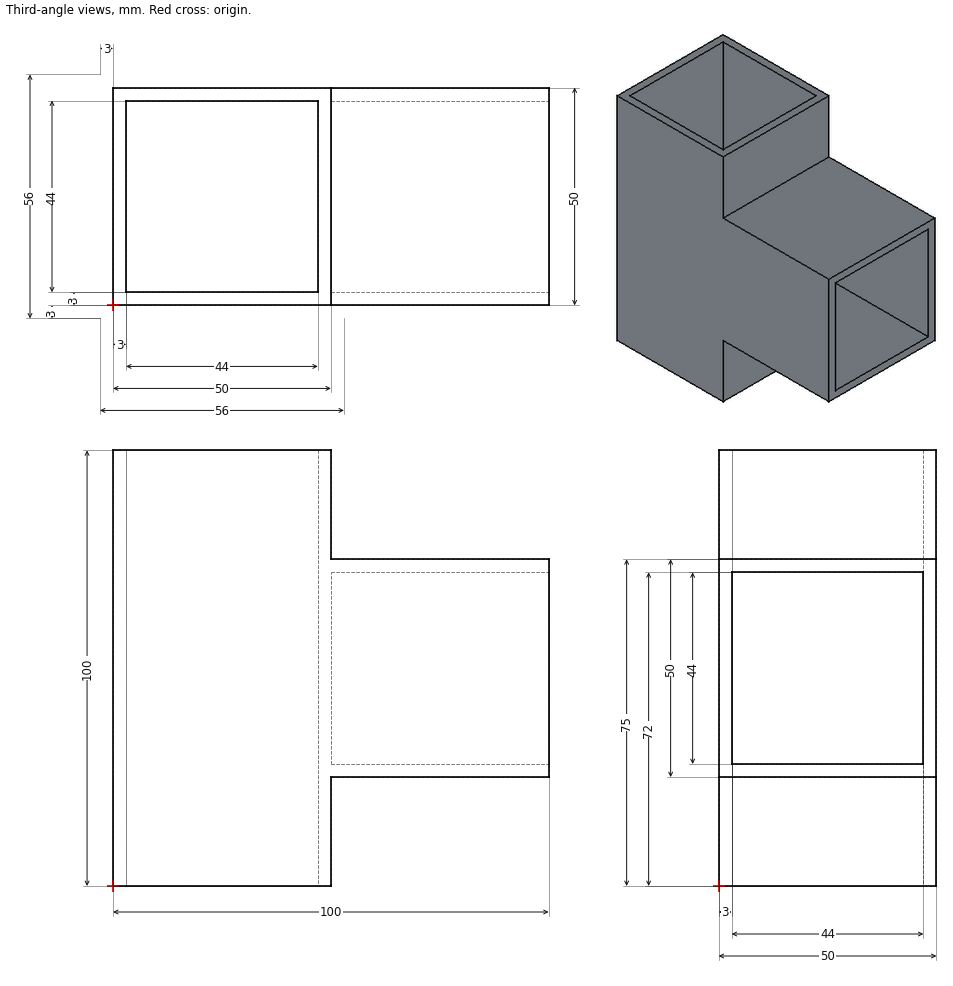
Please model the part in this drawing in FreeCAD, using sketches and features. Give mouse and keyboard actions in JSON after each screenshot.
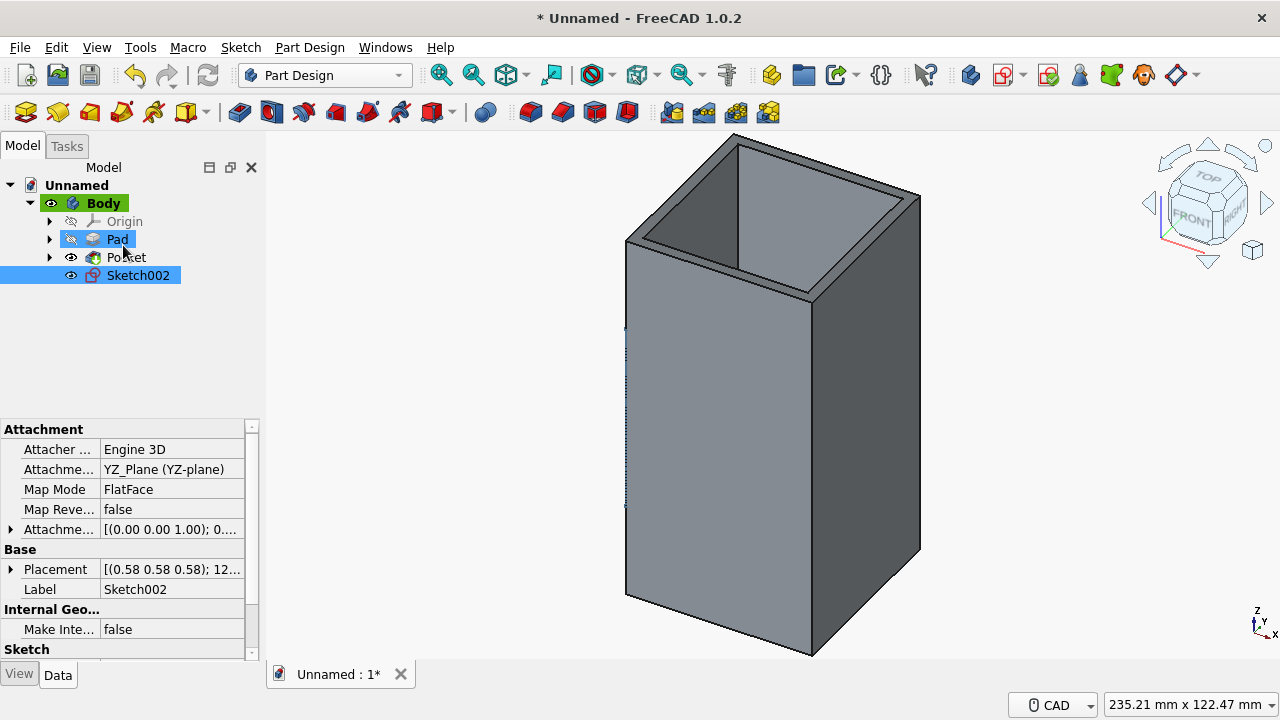
{"action": "left_click", "coordinate": [26, 112]}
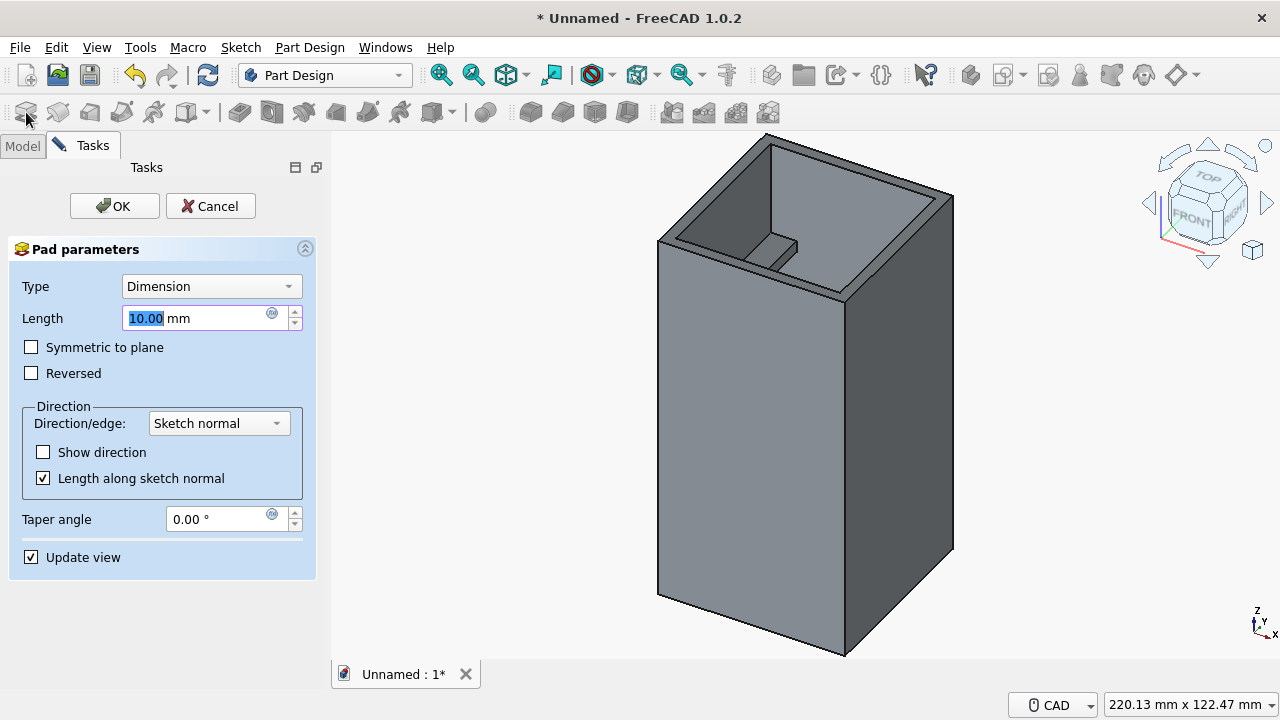
{"action": "type", "text": "100"}
{"action": "key", "text": "Tab"}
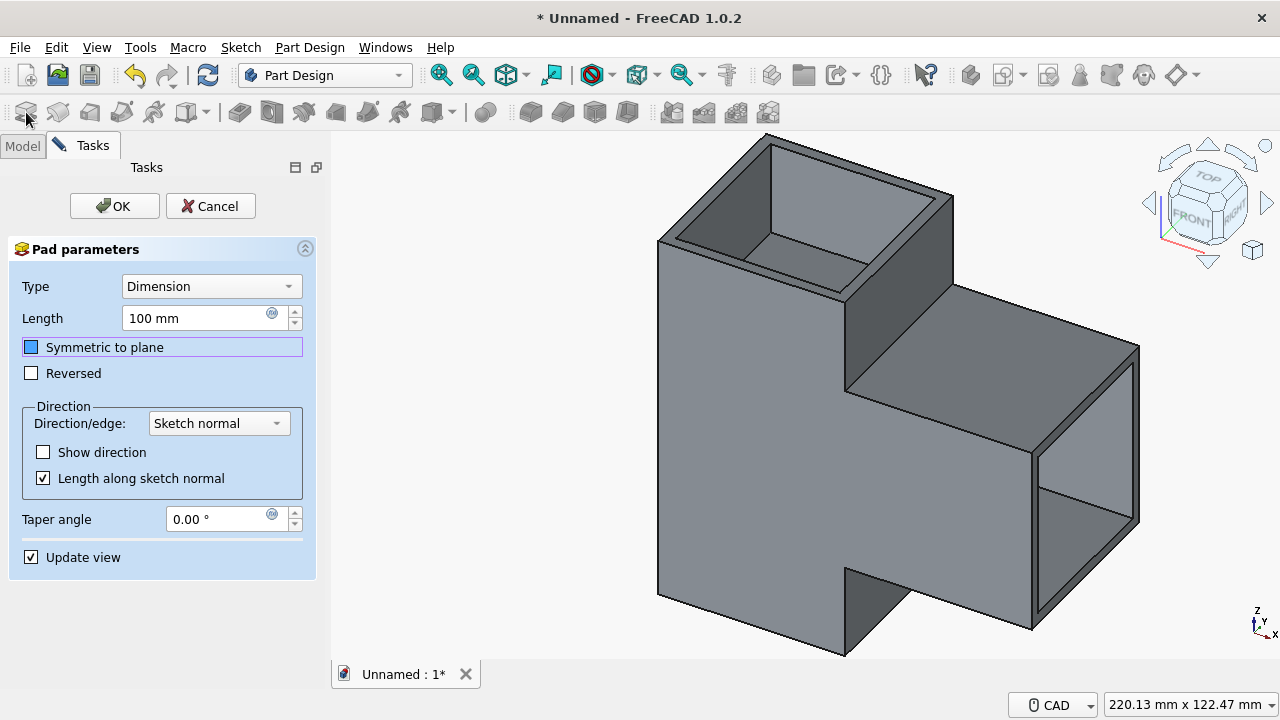
{"action": "left_click", "coordinate": [115, 206]}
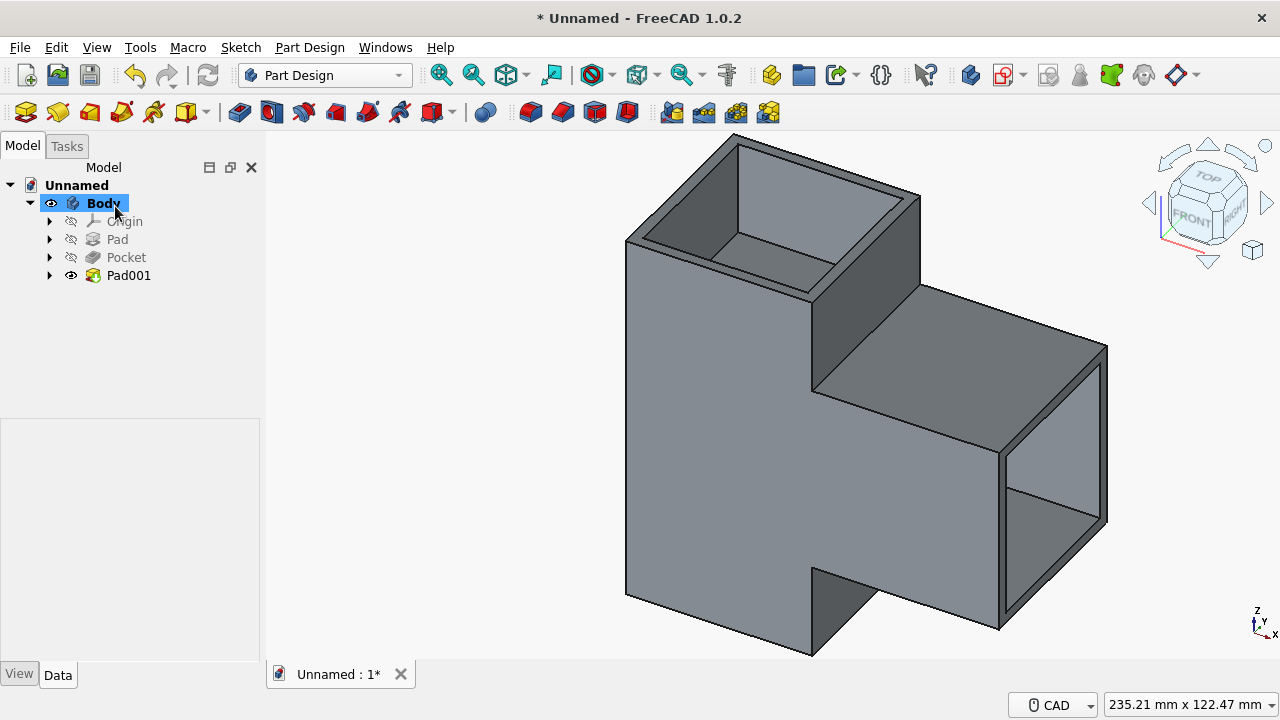
{"action": "left_click", "coordinate": [442, 76]}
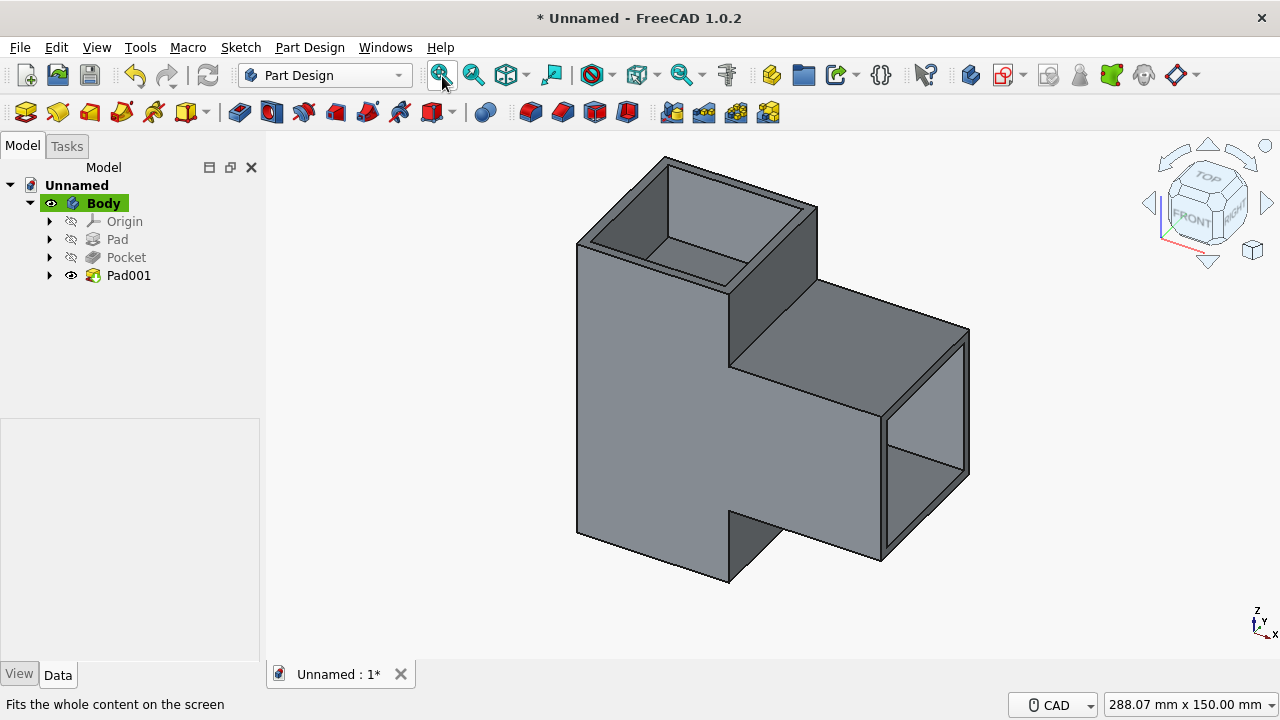
{"action": "key", "text": "5"}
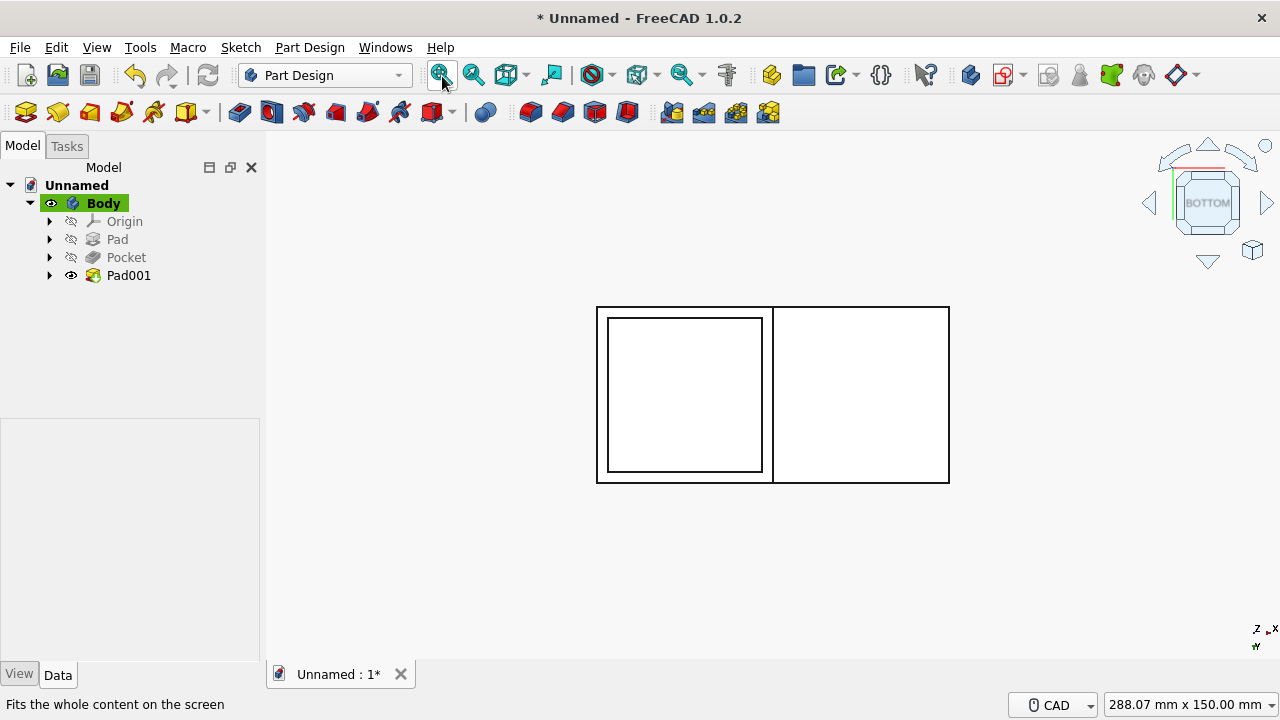
{"action": "left_click", "coordinate": [442, 76]}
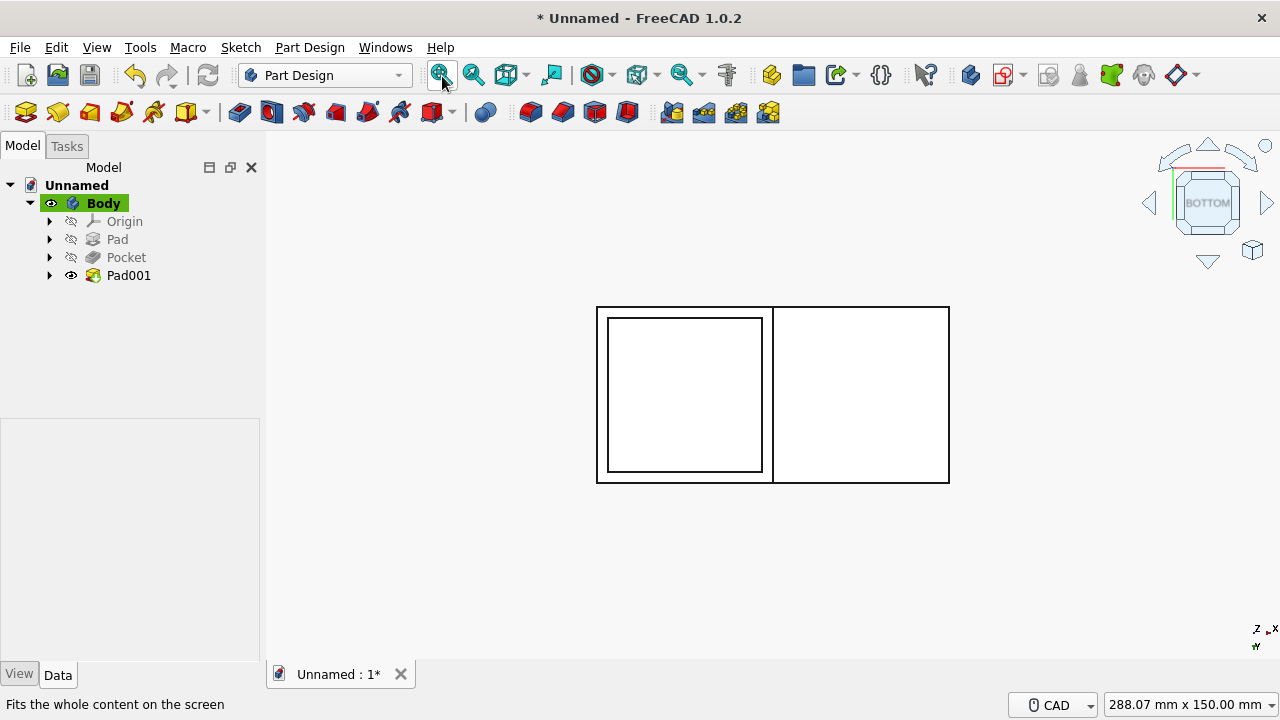
{"action": "scroll", "coordinate": [769, 368], "scroll_direction": "up", "scroll_amount": 7}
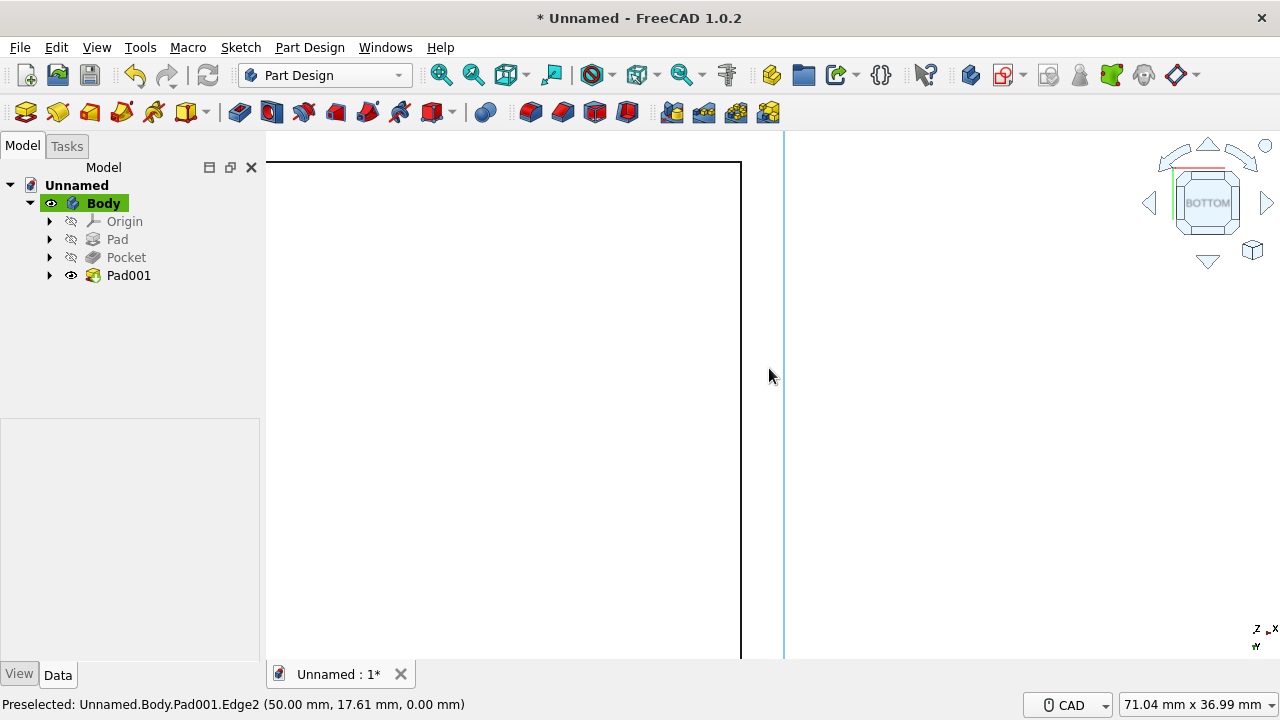
{"action": "left_click", "coordinate": [769, 370]}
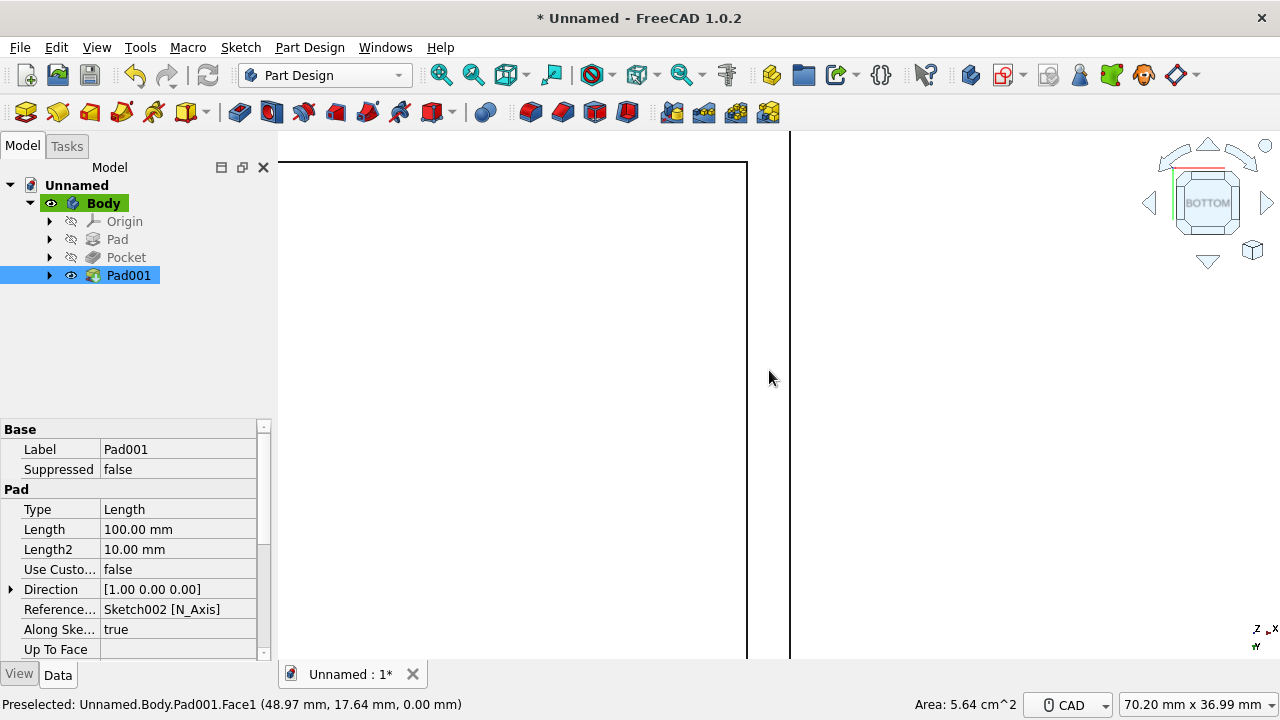
{"action": "left_click", "coordinate": [1004, 76]}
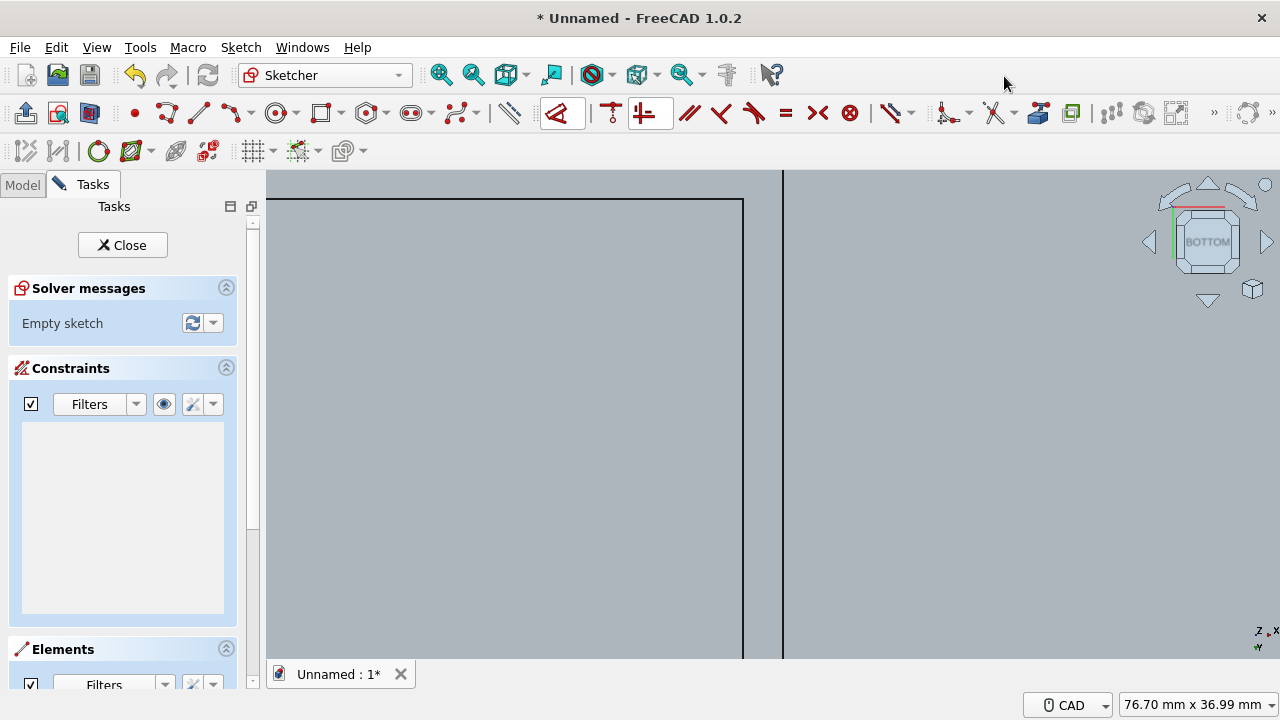
{"action": "scroll", "coordinate": [926, 369], "scroll_direction": "down", "scroll_amount": 4}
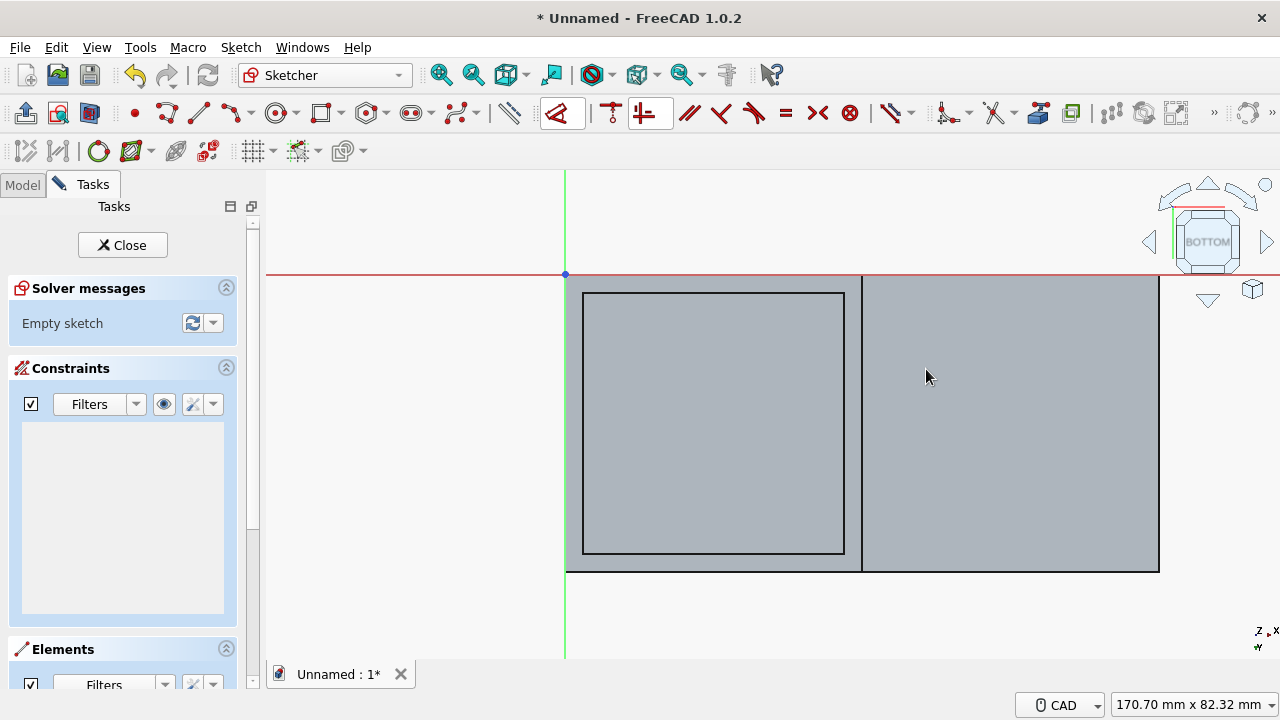
{"action": "key", "text": "g r"}